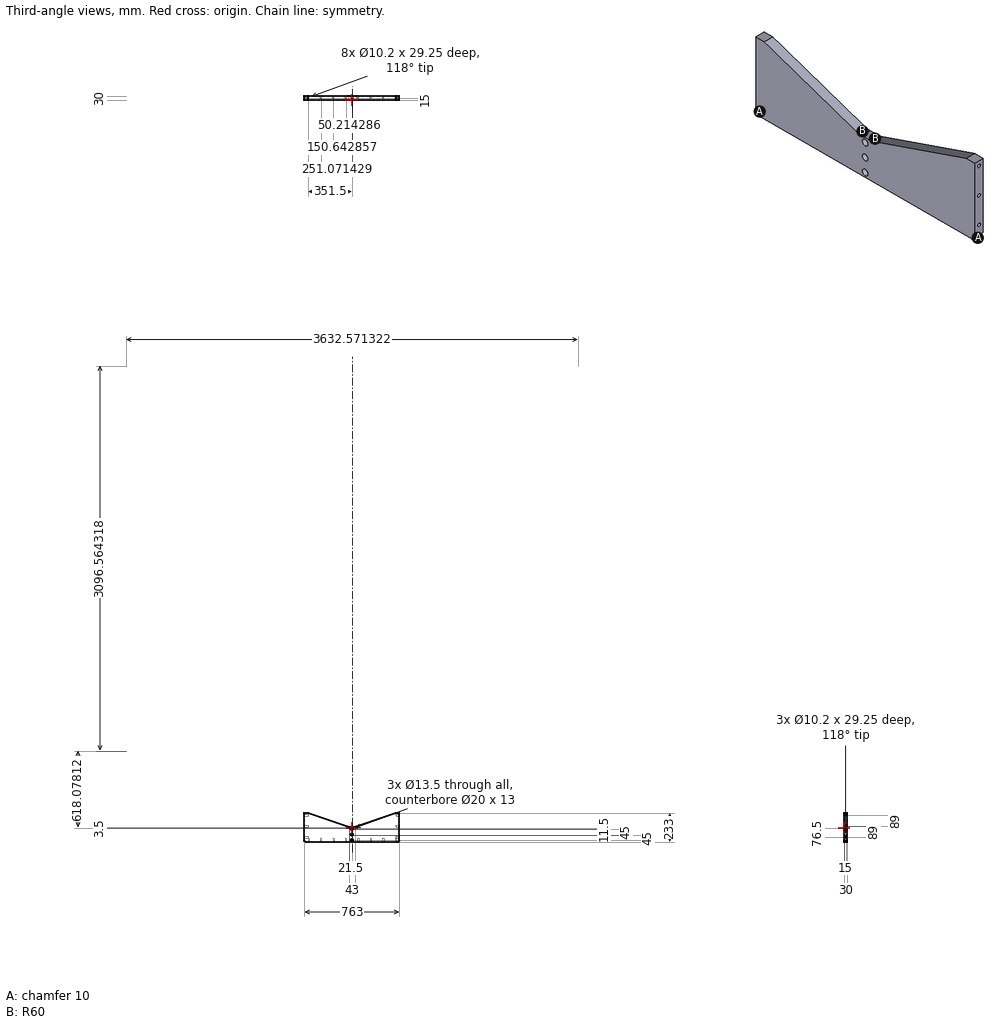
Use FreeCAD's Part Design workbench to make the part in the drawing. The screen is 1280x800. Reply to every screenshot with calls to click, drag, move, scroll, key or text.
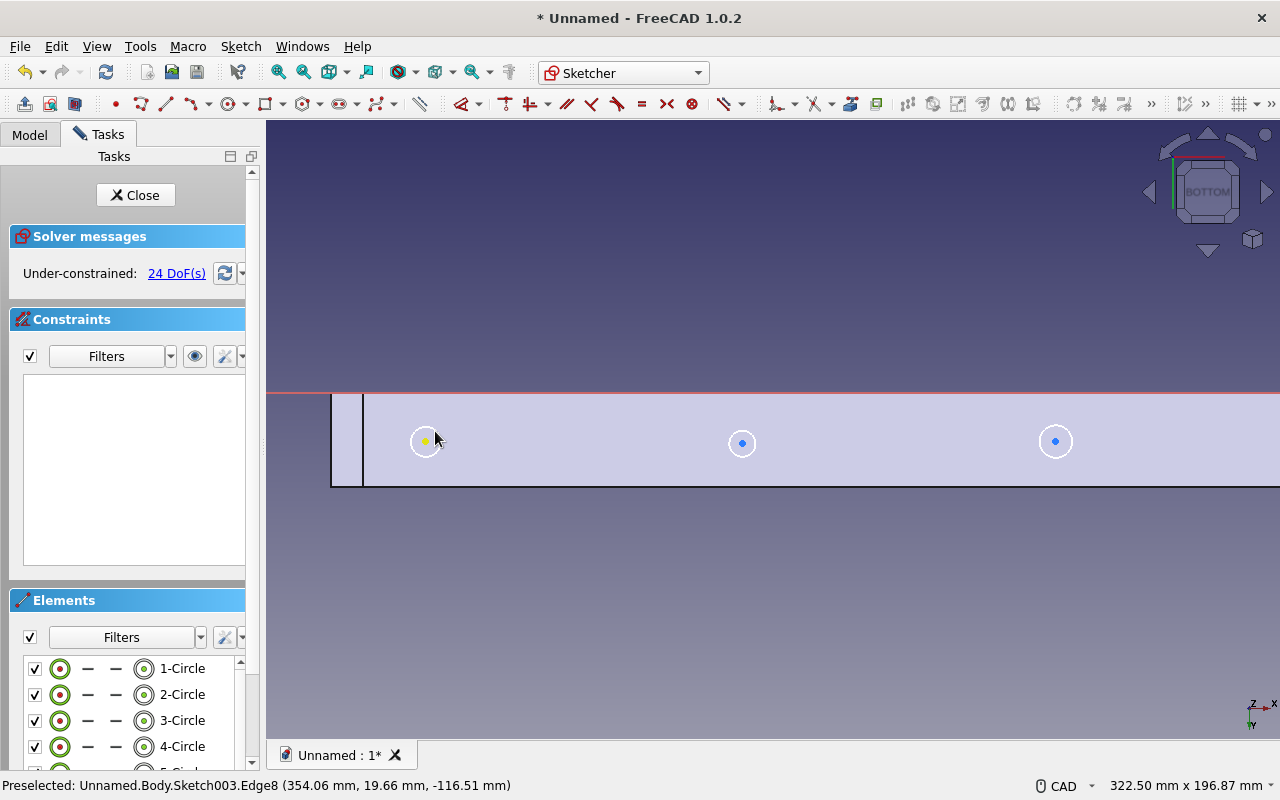
click(436, 431)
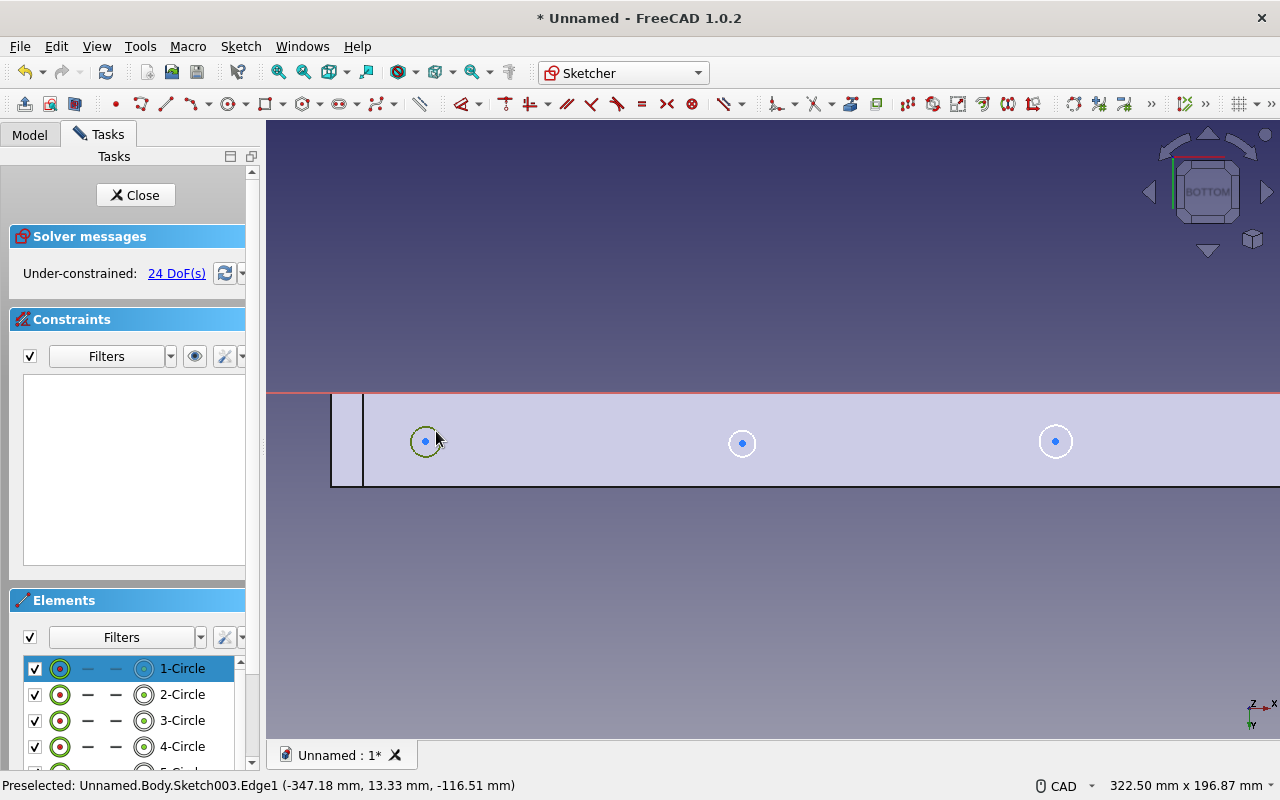
click(752, 434)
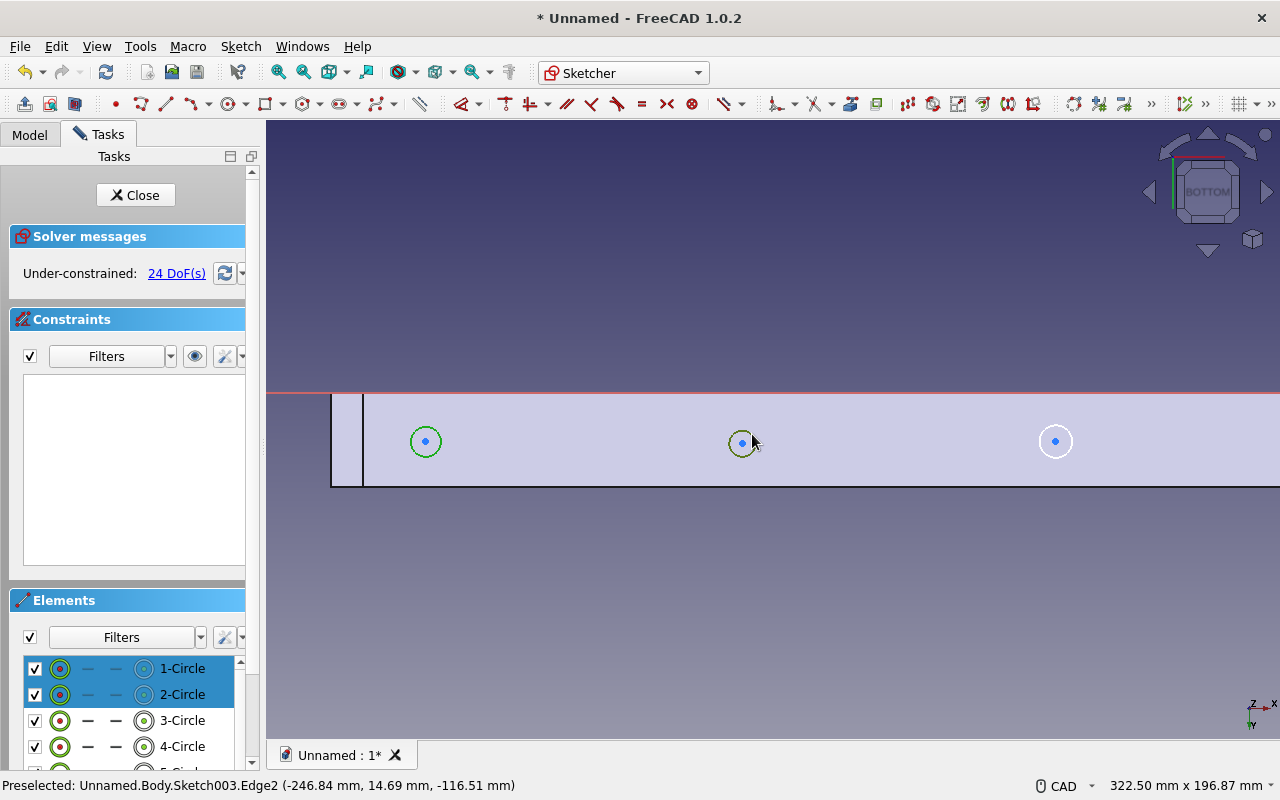
click(1067, 430)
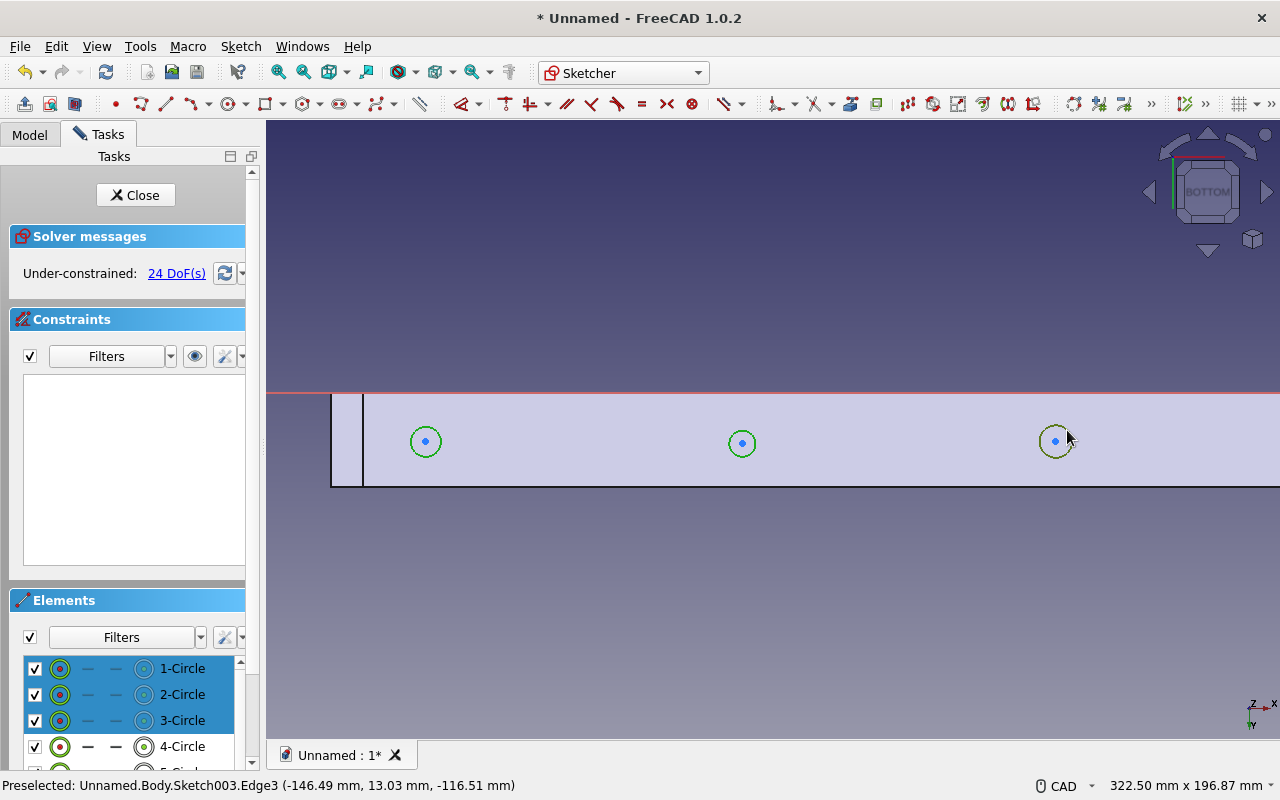
scroll(434, 431, down, 7)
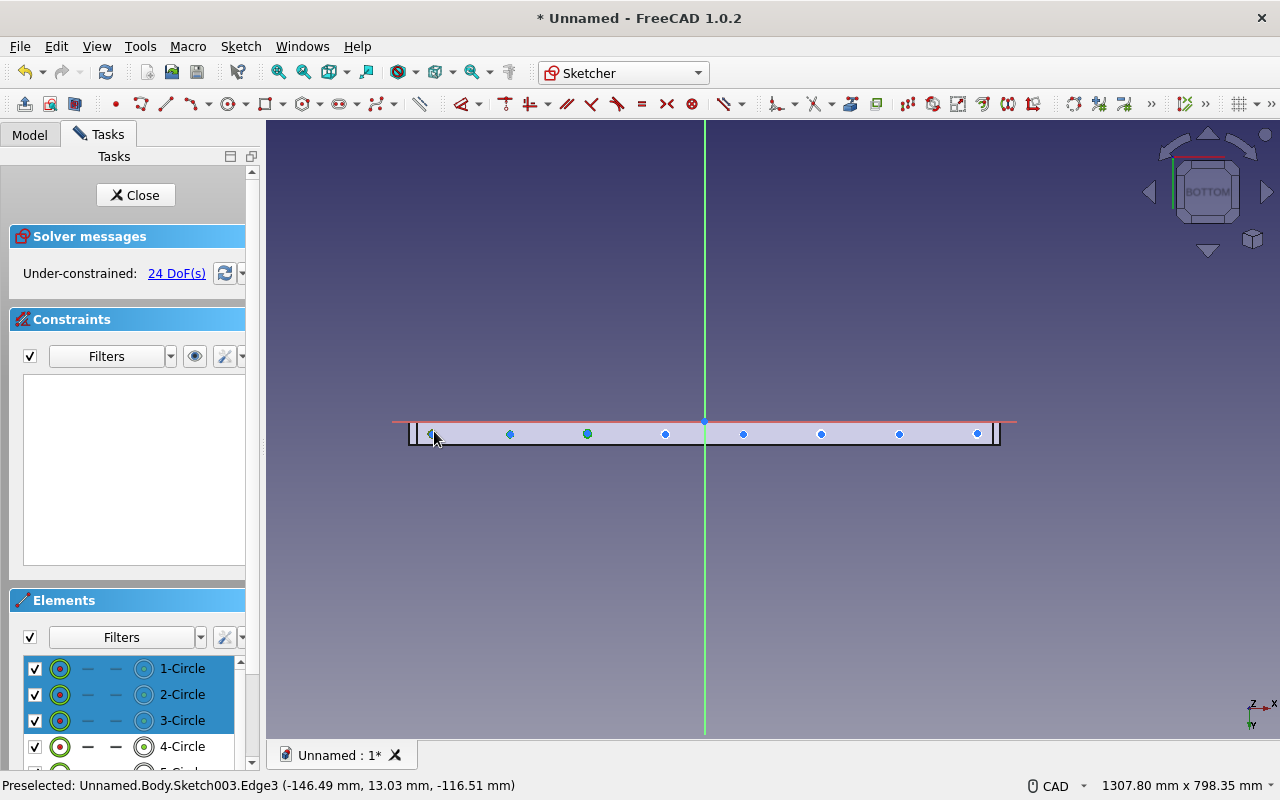
scroll(668, 431, up, 7)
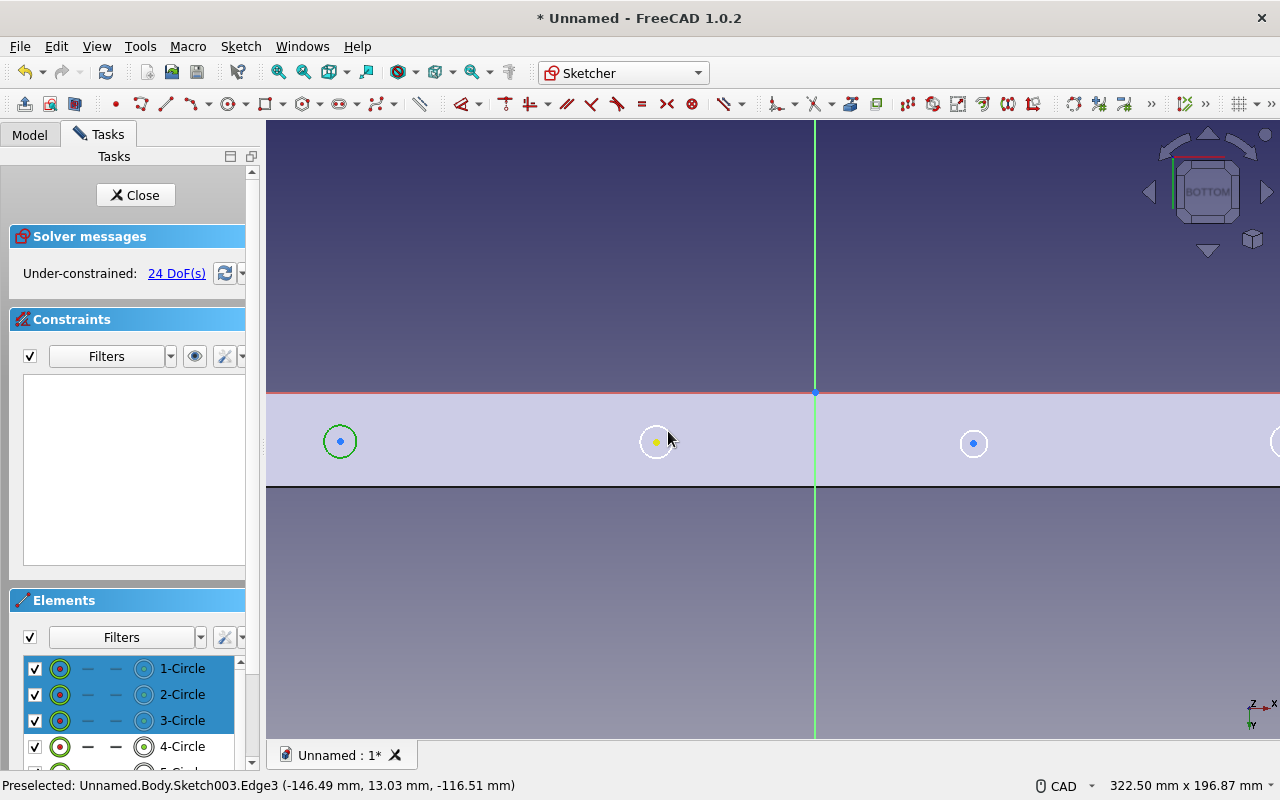
click(668, 431)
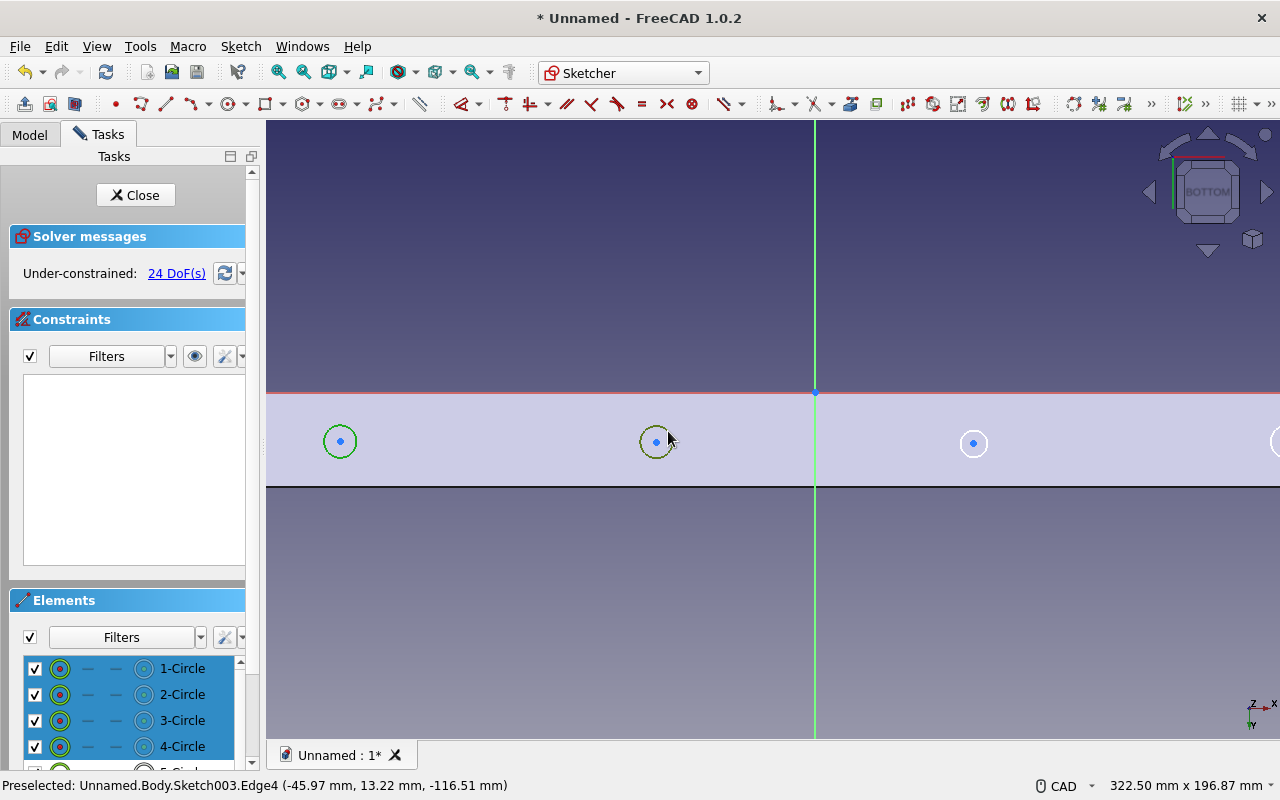
click(983, 434)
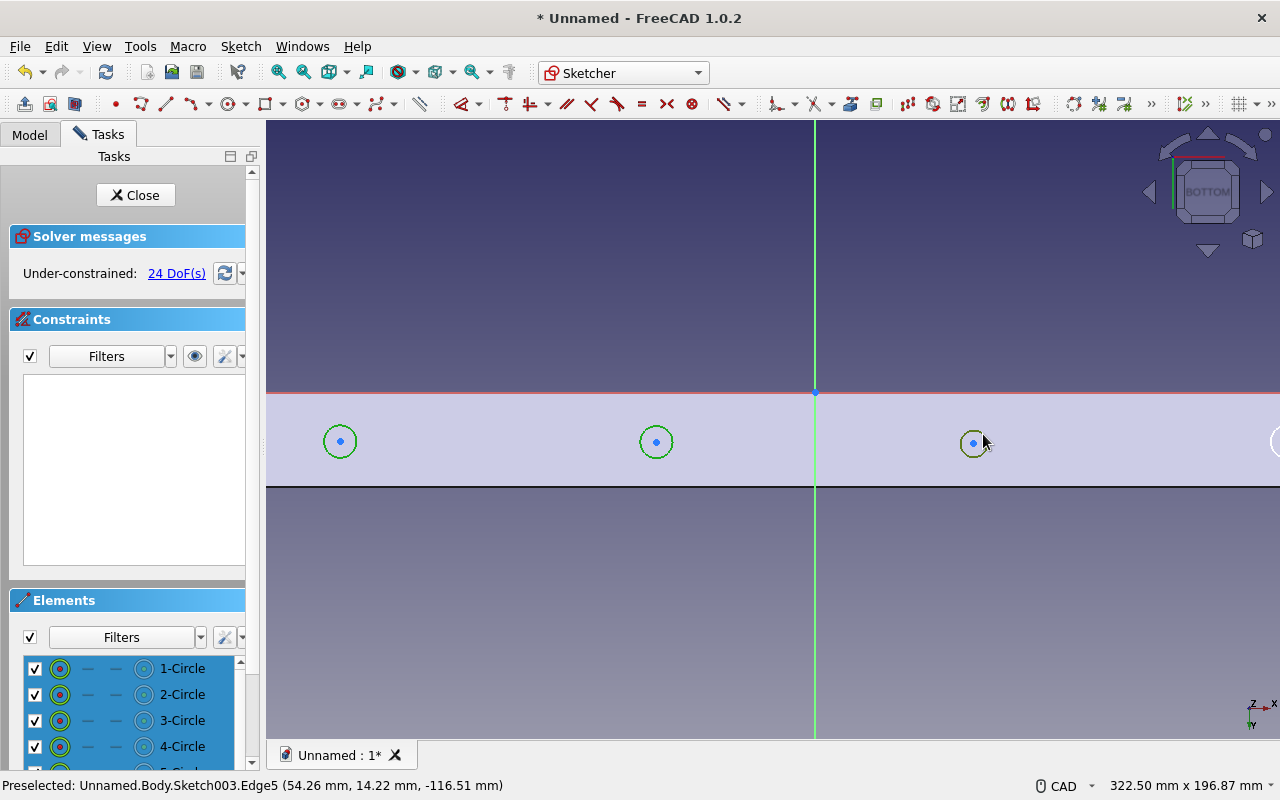
scroll(668, 431, down, 7)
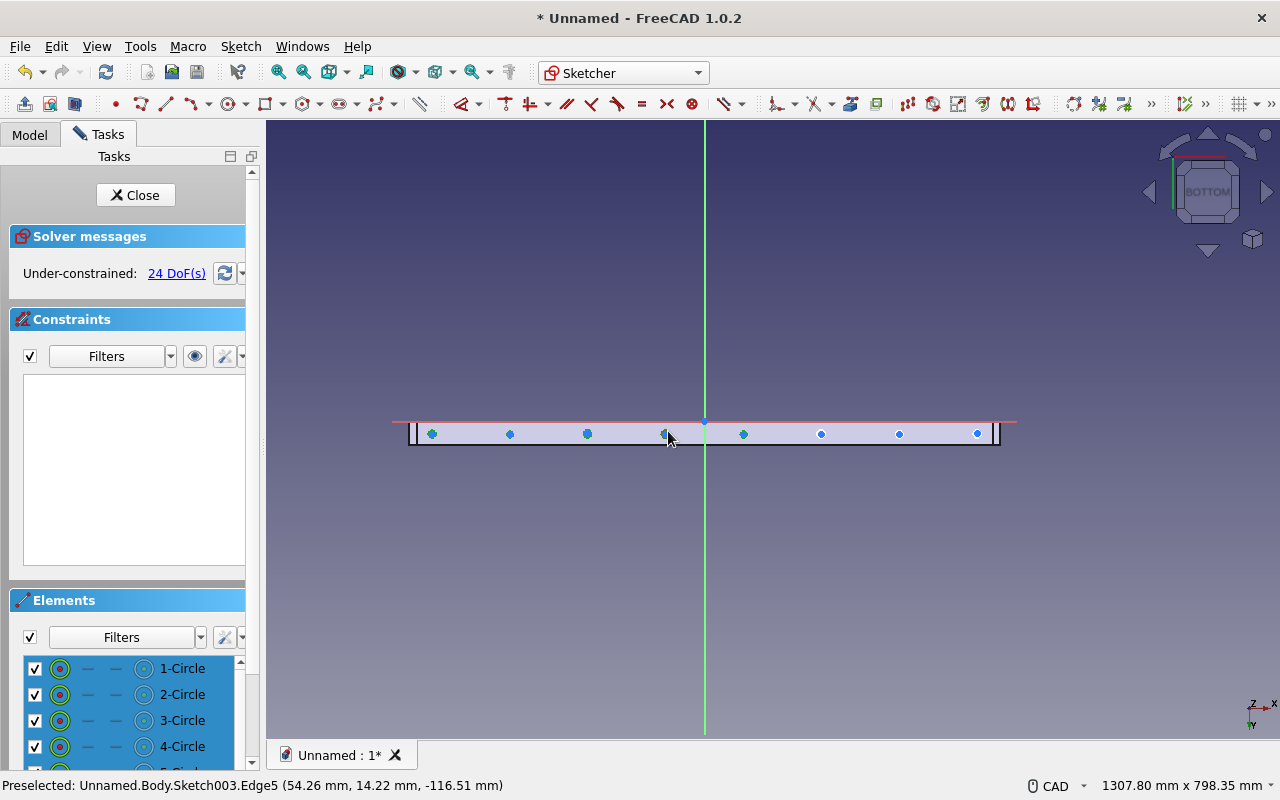
scroll(824, 431, up, 7)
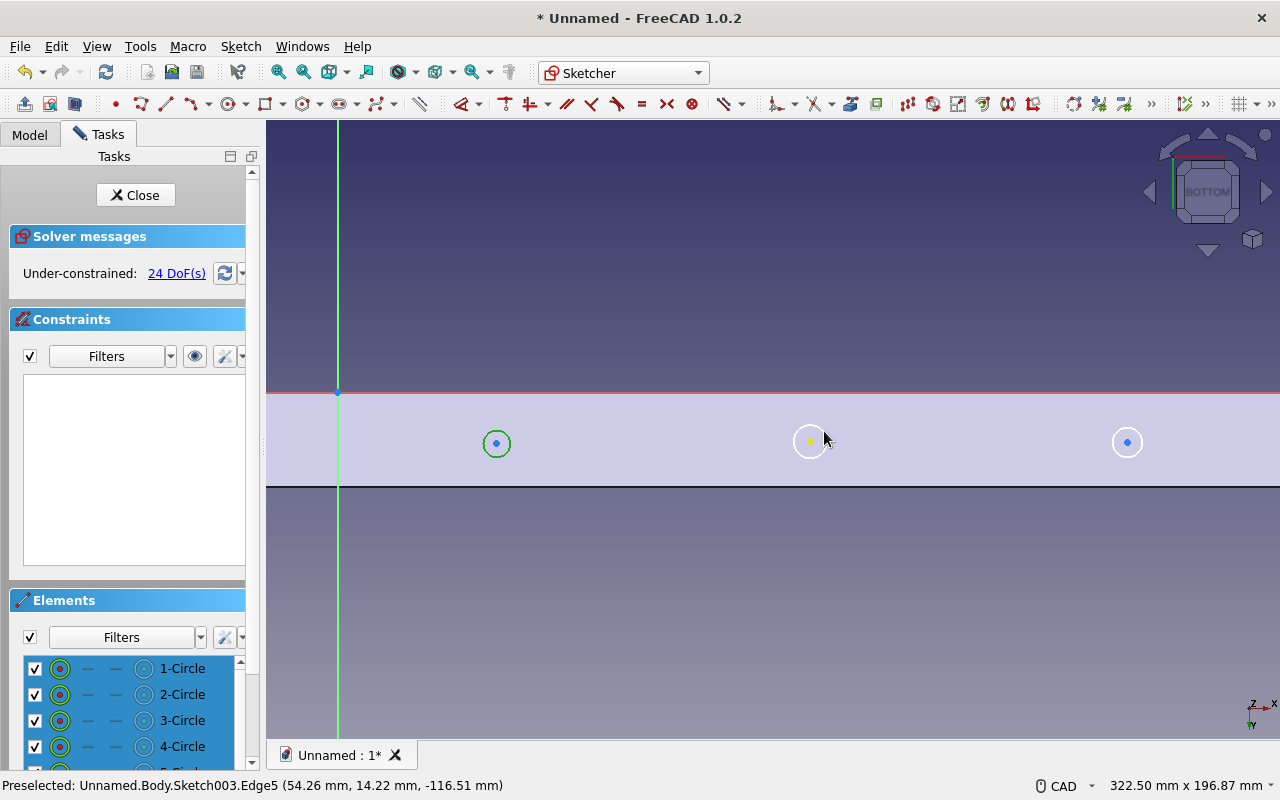
click(822, 430)